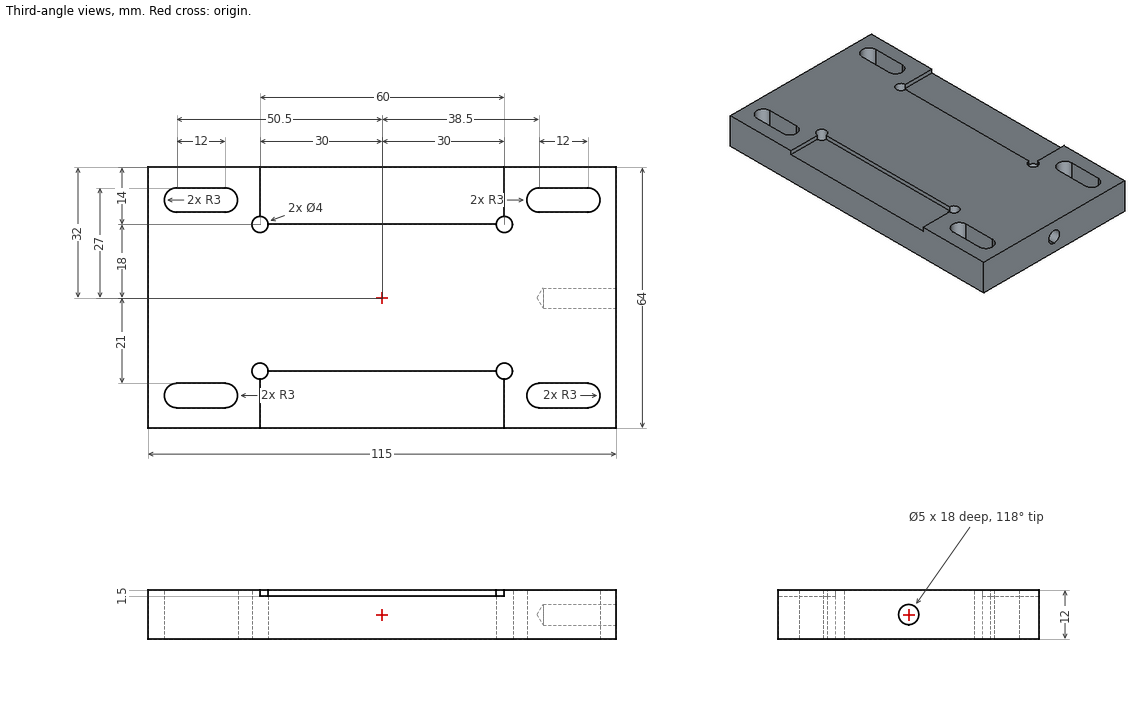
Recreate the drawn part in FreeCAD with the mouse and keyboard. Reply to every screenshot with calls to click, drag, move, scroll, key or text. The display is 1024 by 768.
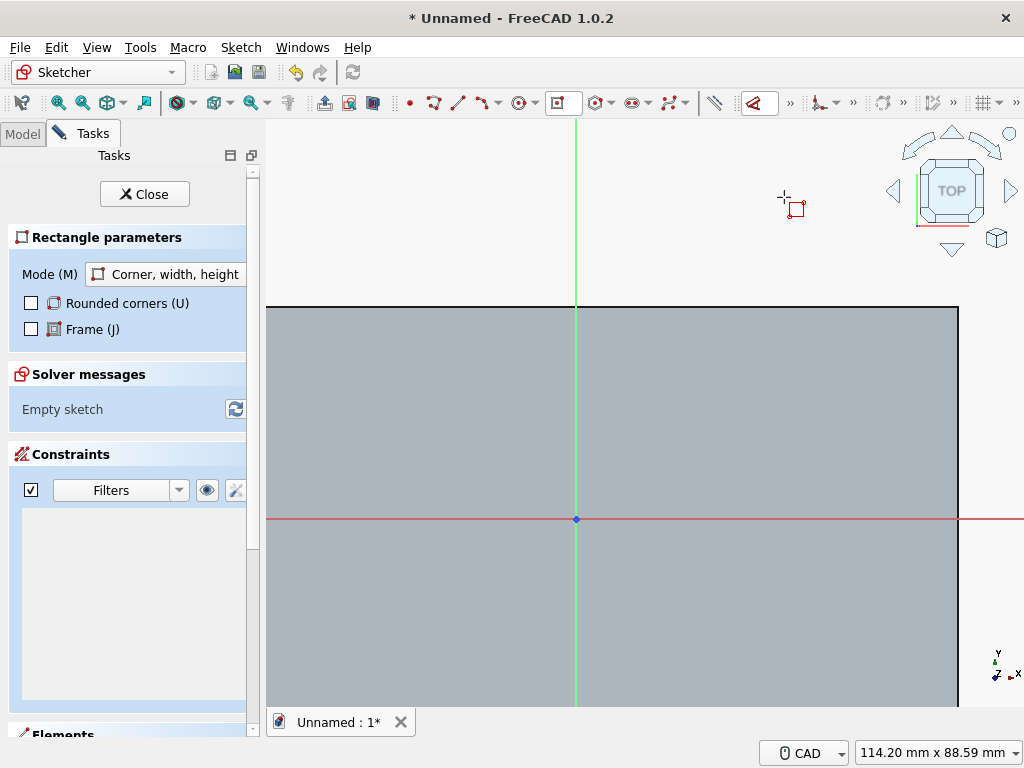
click(377, 307)
click(775, 400)
key(Escape)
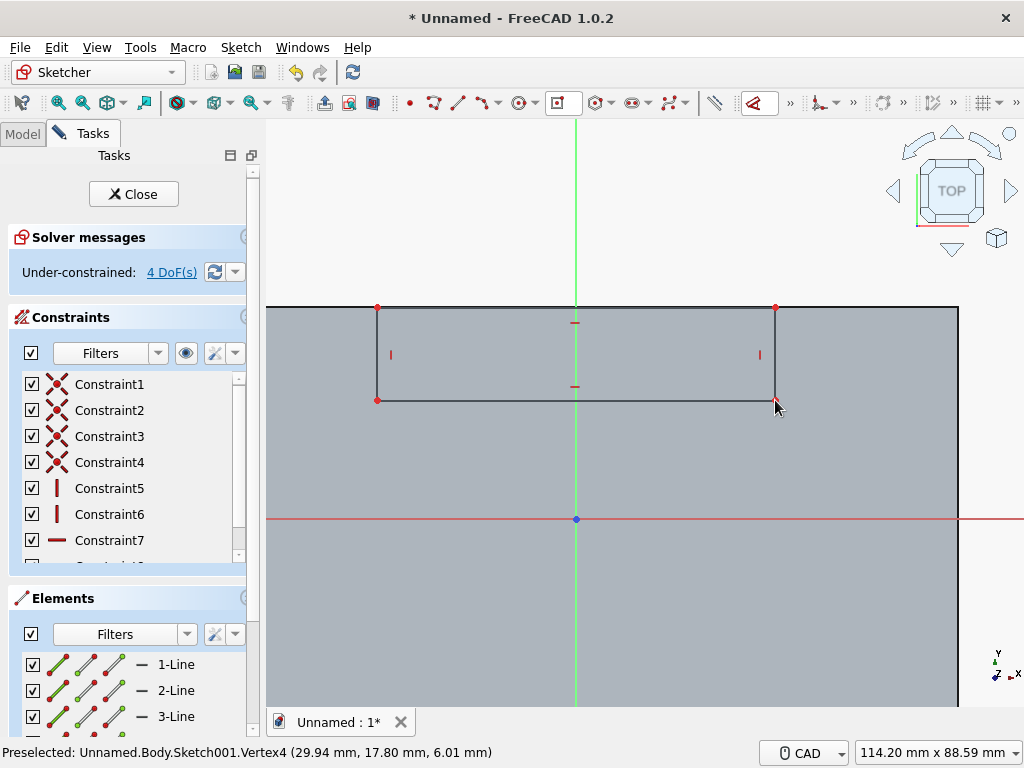
click(377, 336)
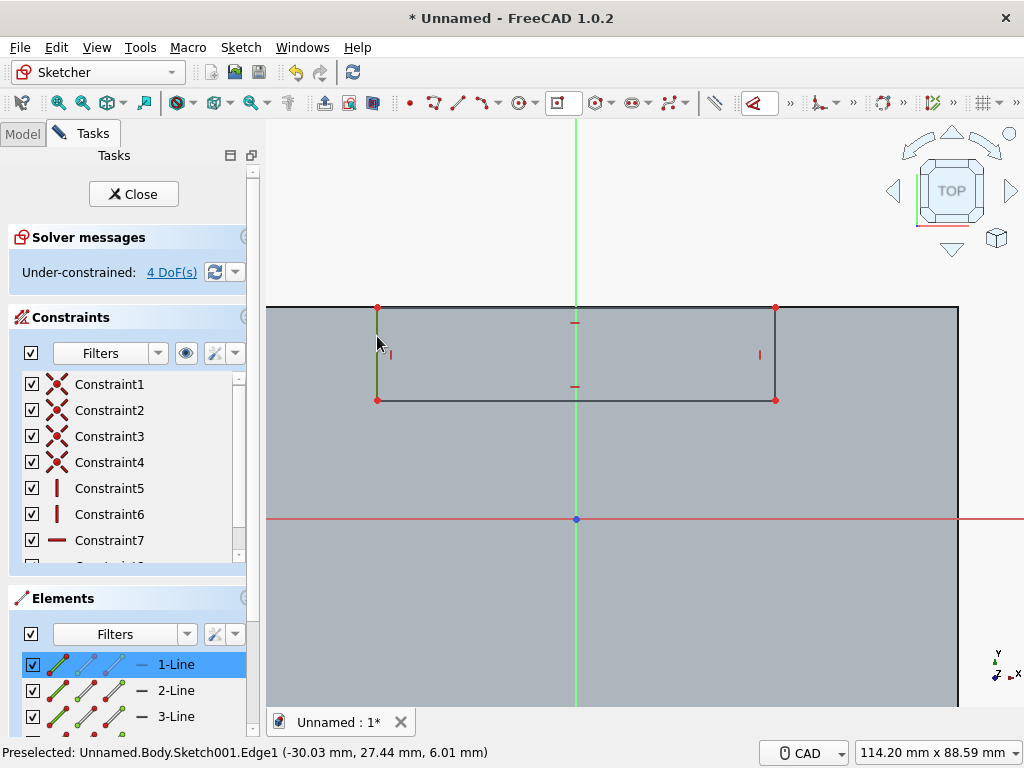
key(i)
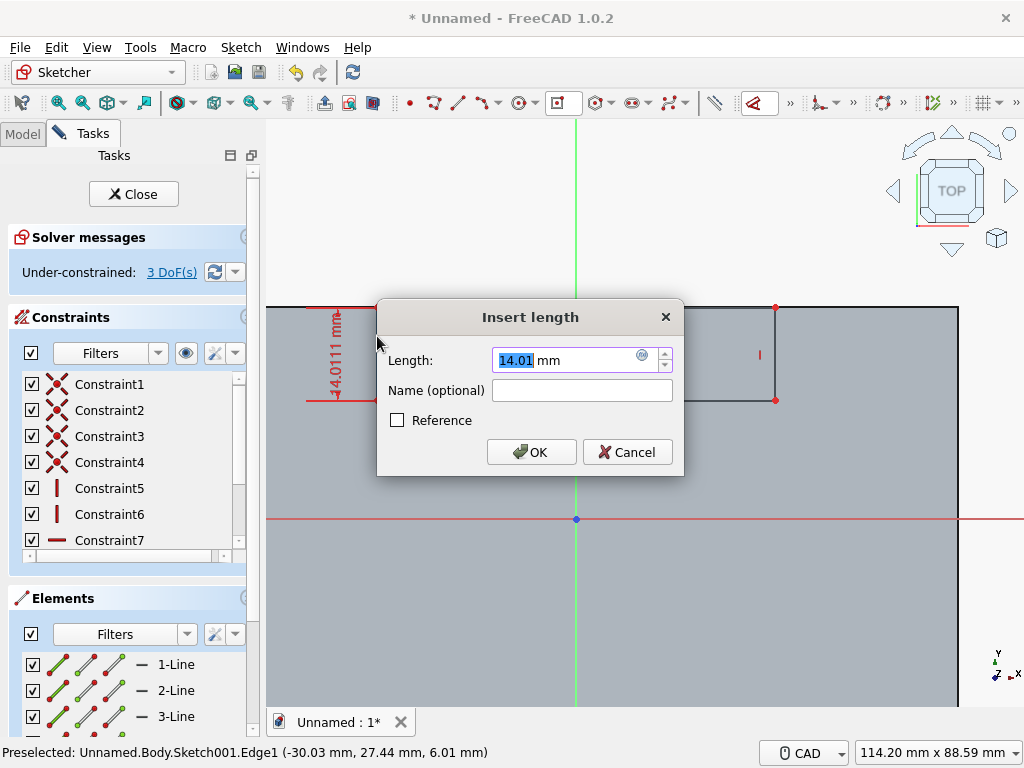
text(14)
key(Return)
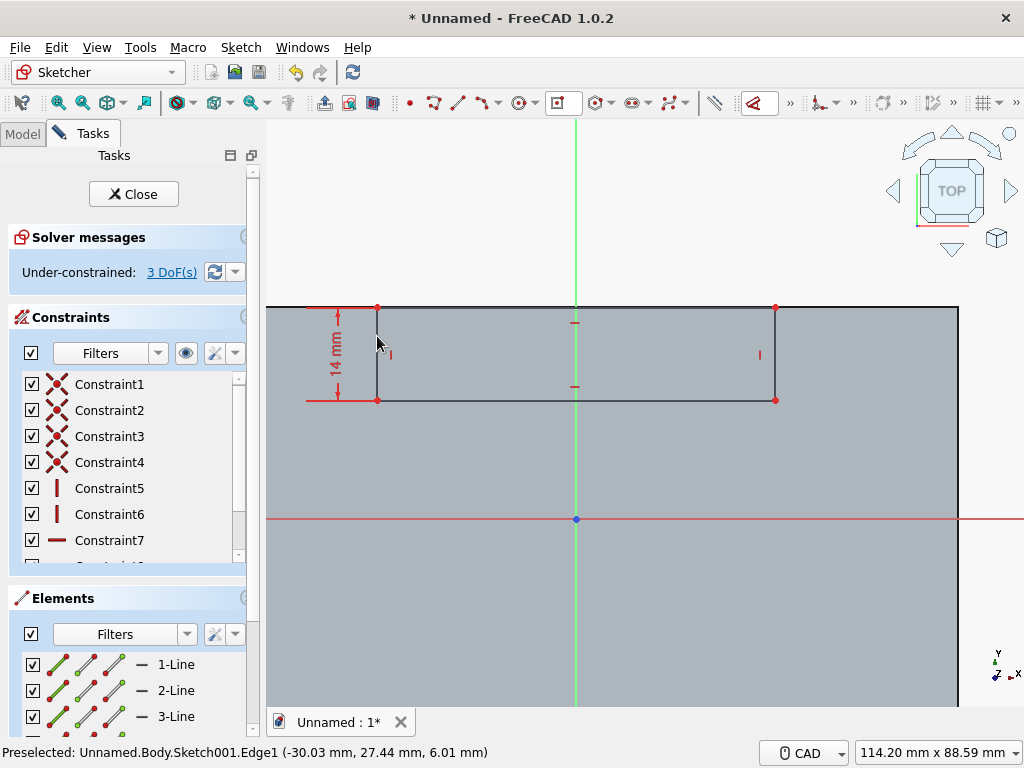
click(496, 401)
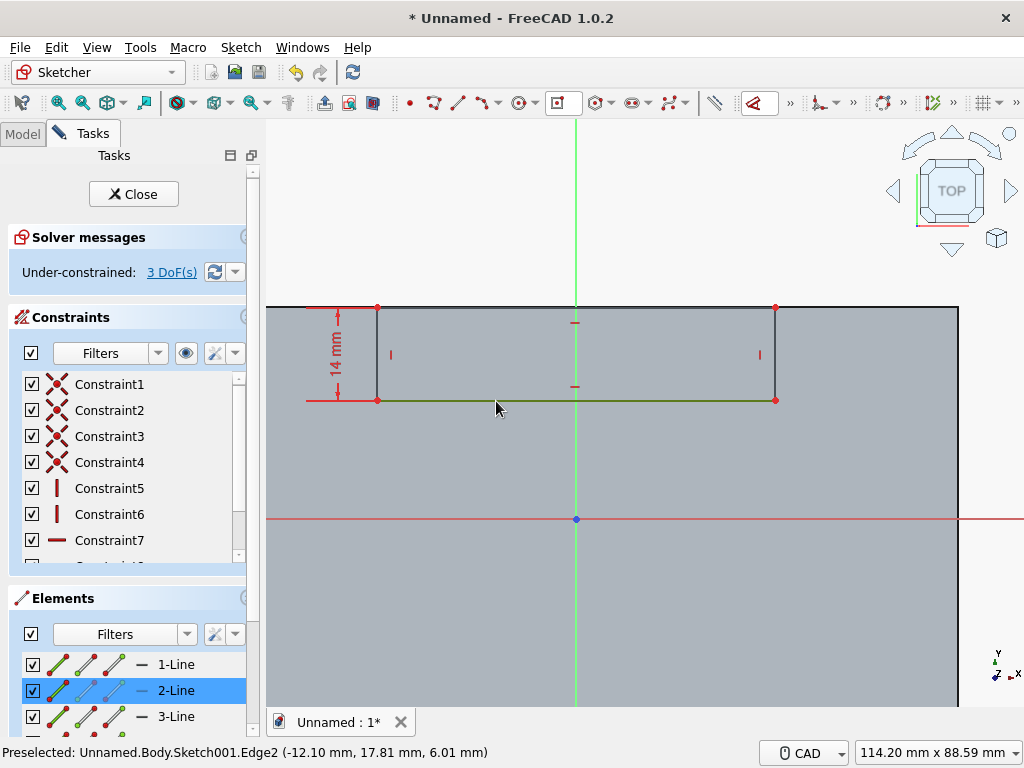
key(l)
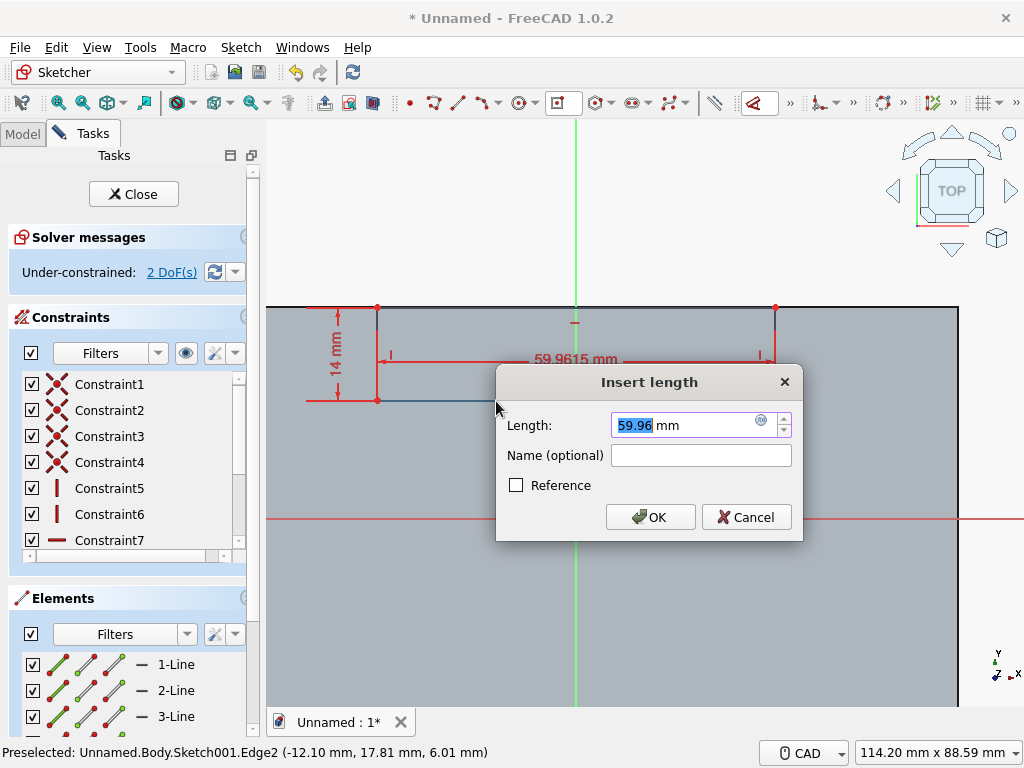
text(60)
key(Return)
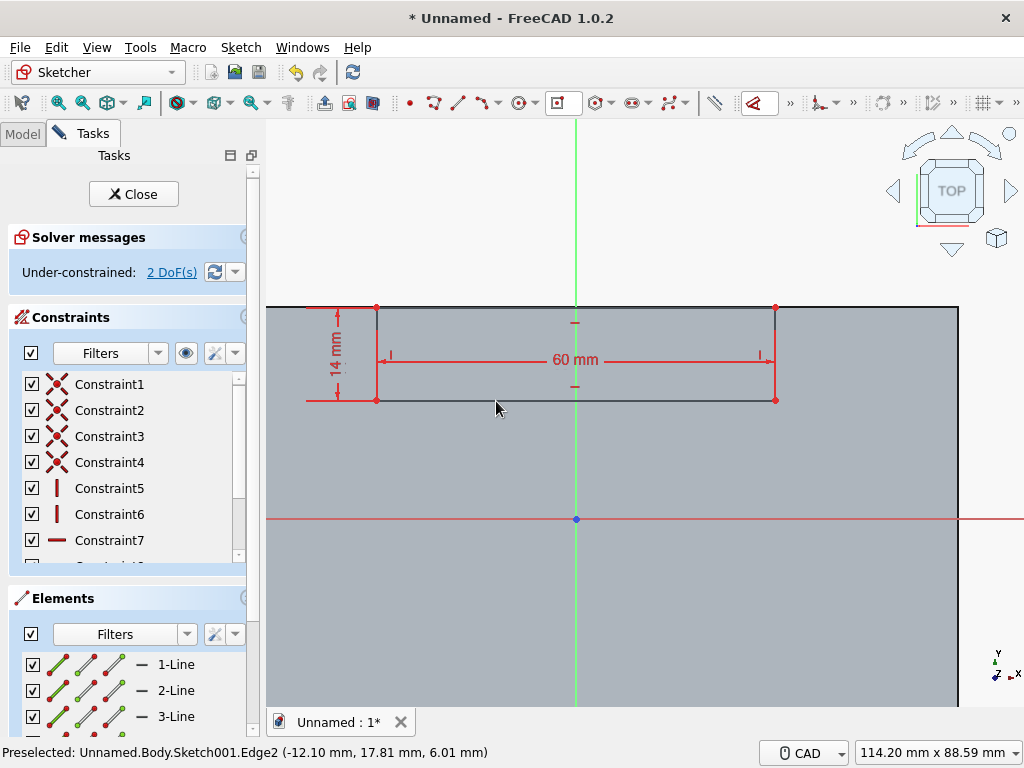
click(377, 308)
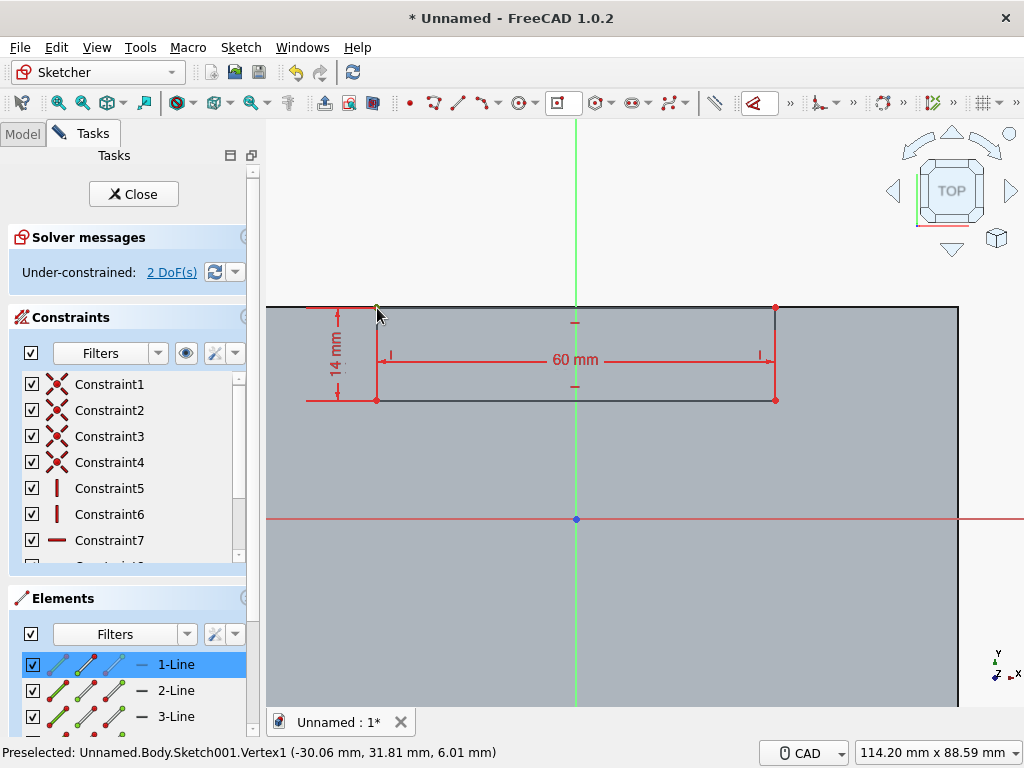
click(772, 104)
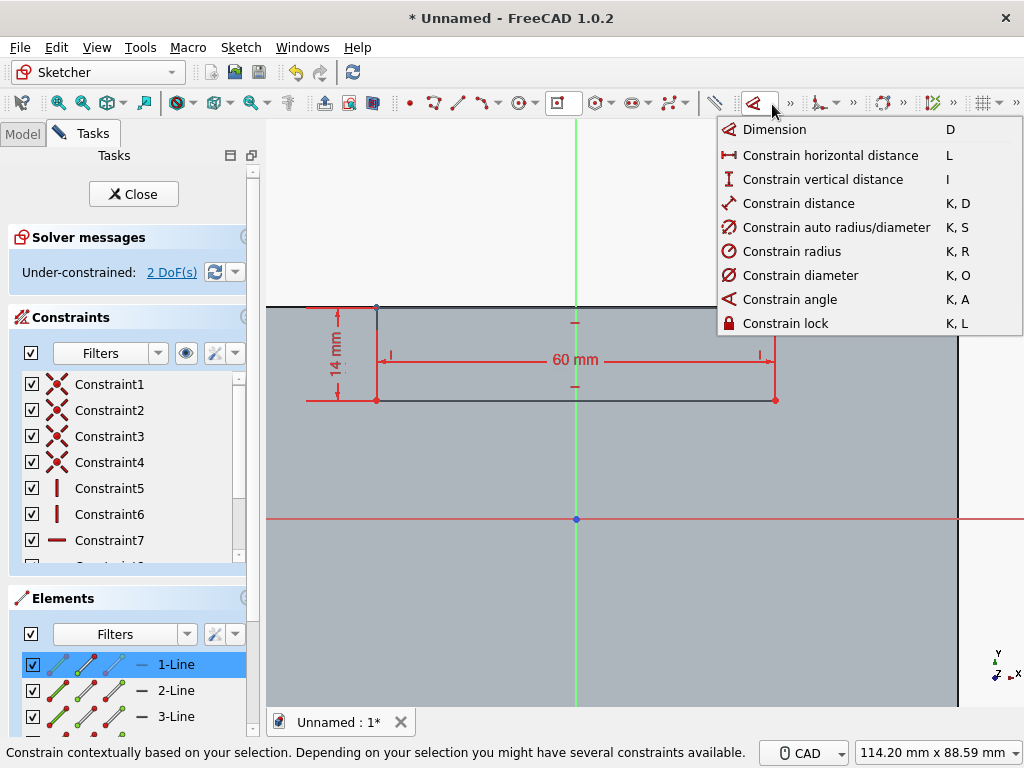
click(870, 155)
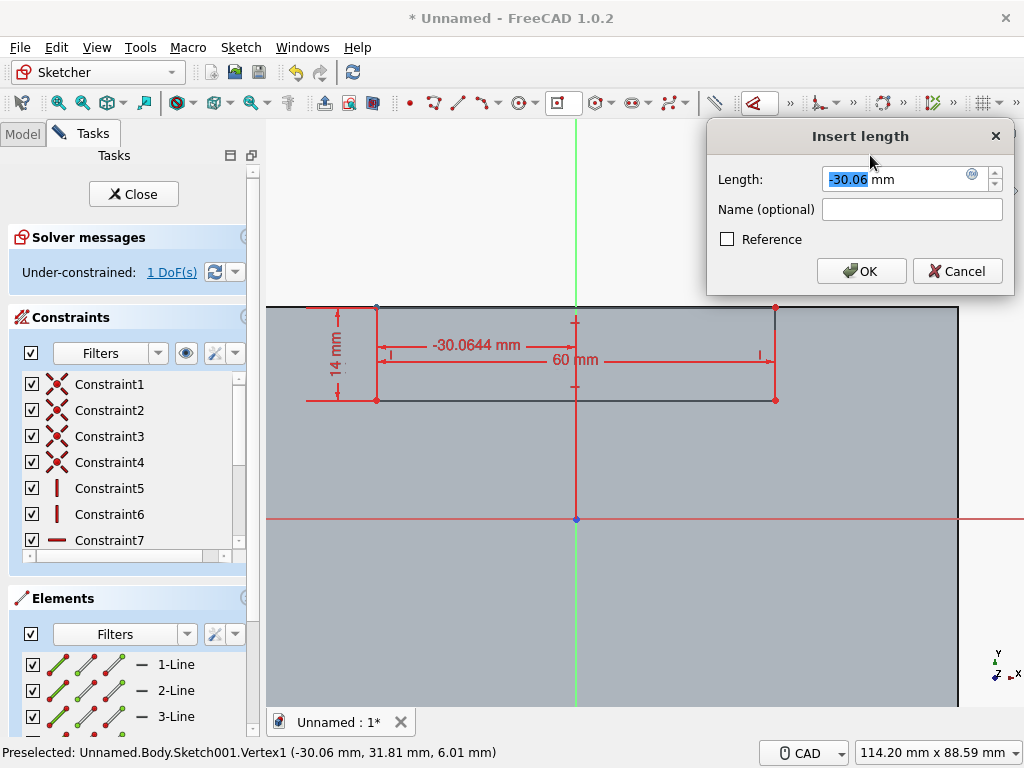
text(-30)
key(Return)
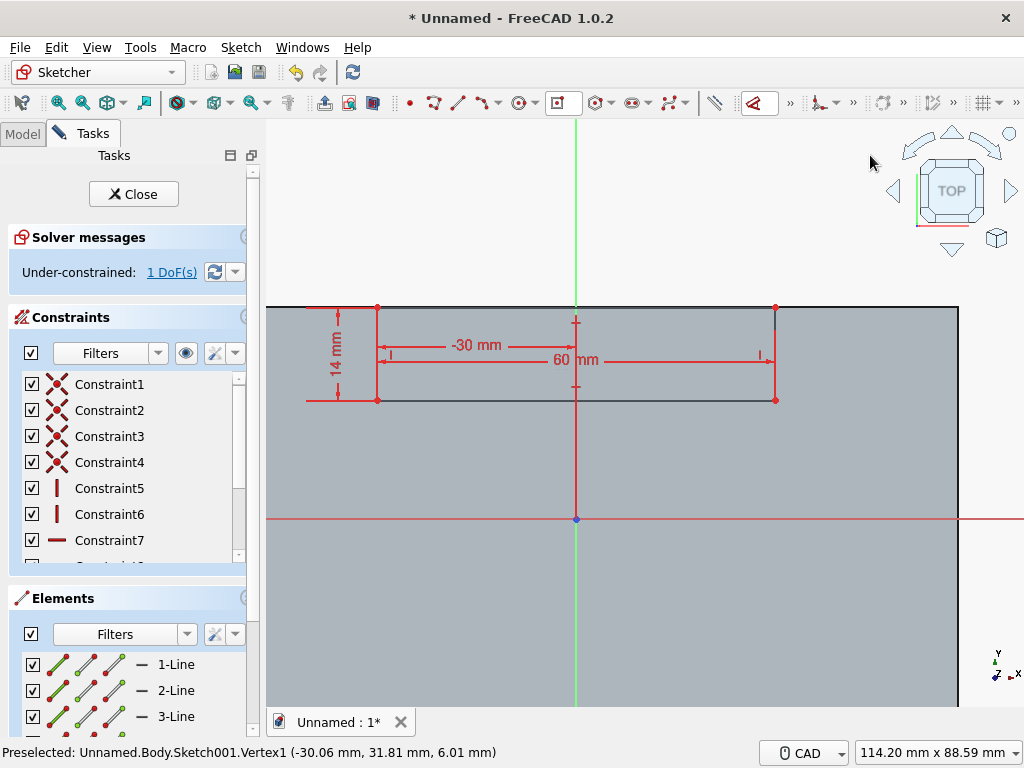
click(377, 308)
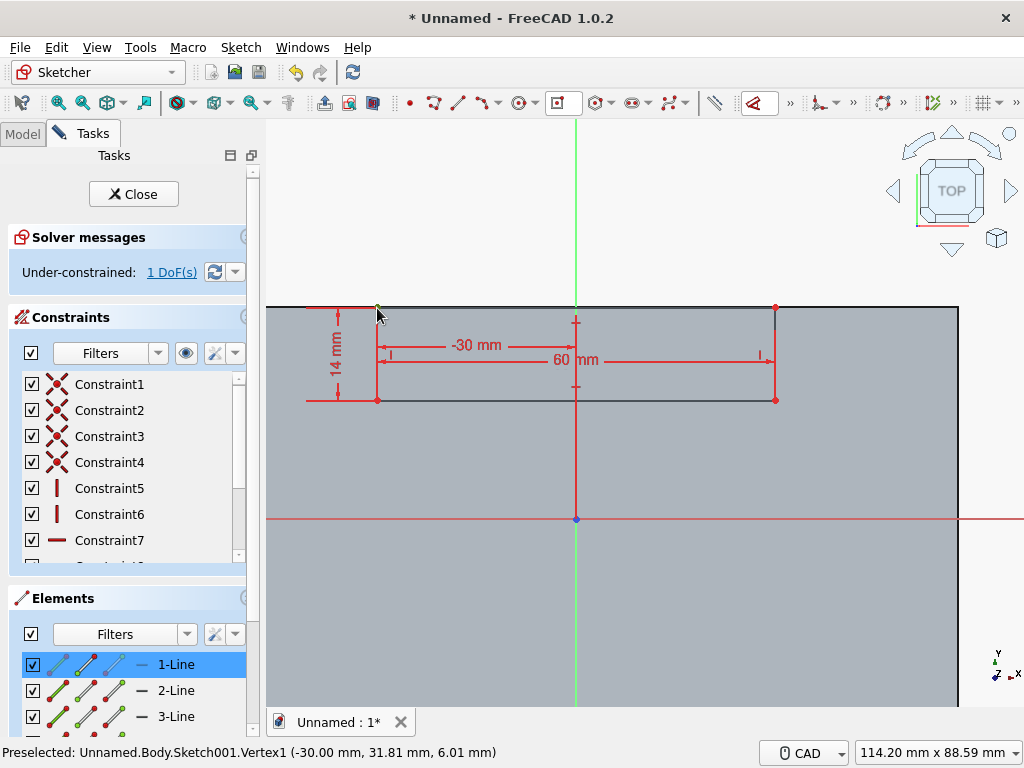
click(772, 104)